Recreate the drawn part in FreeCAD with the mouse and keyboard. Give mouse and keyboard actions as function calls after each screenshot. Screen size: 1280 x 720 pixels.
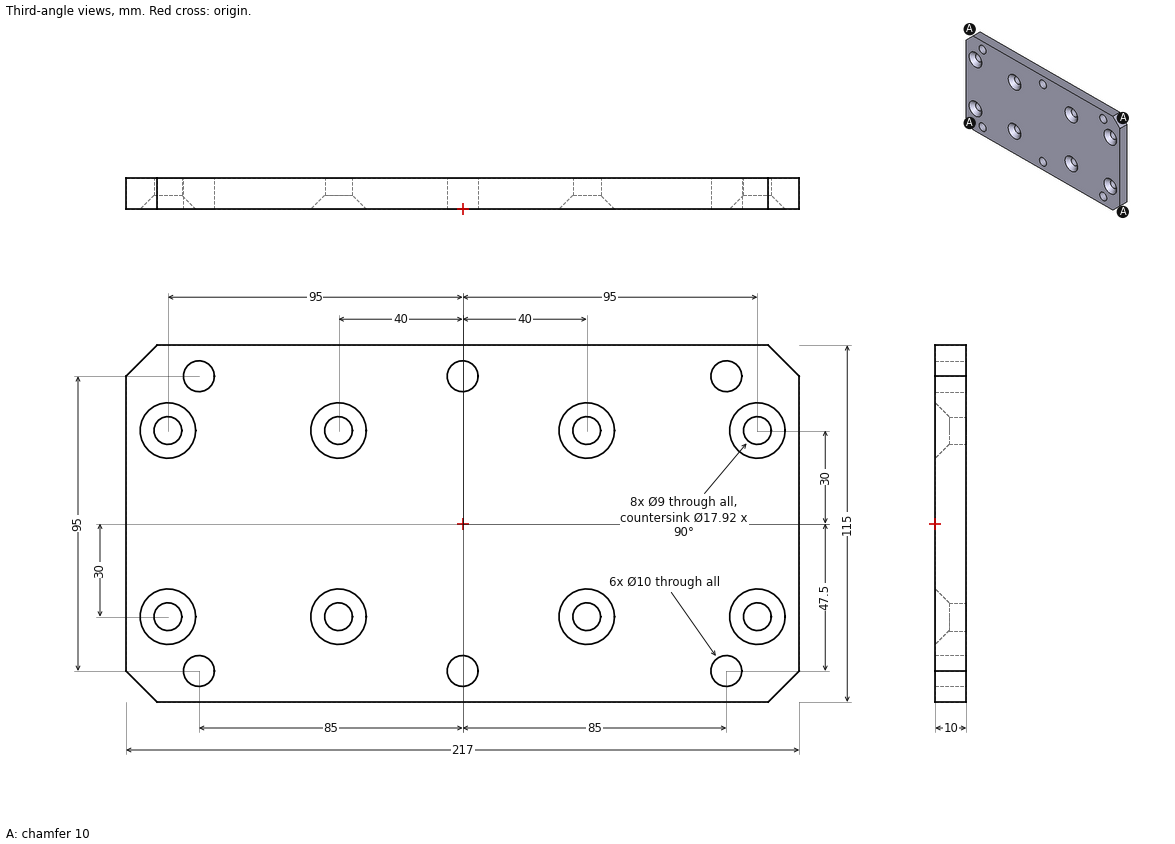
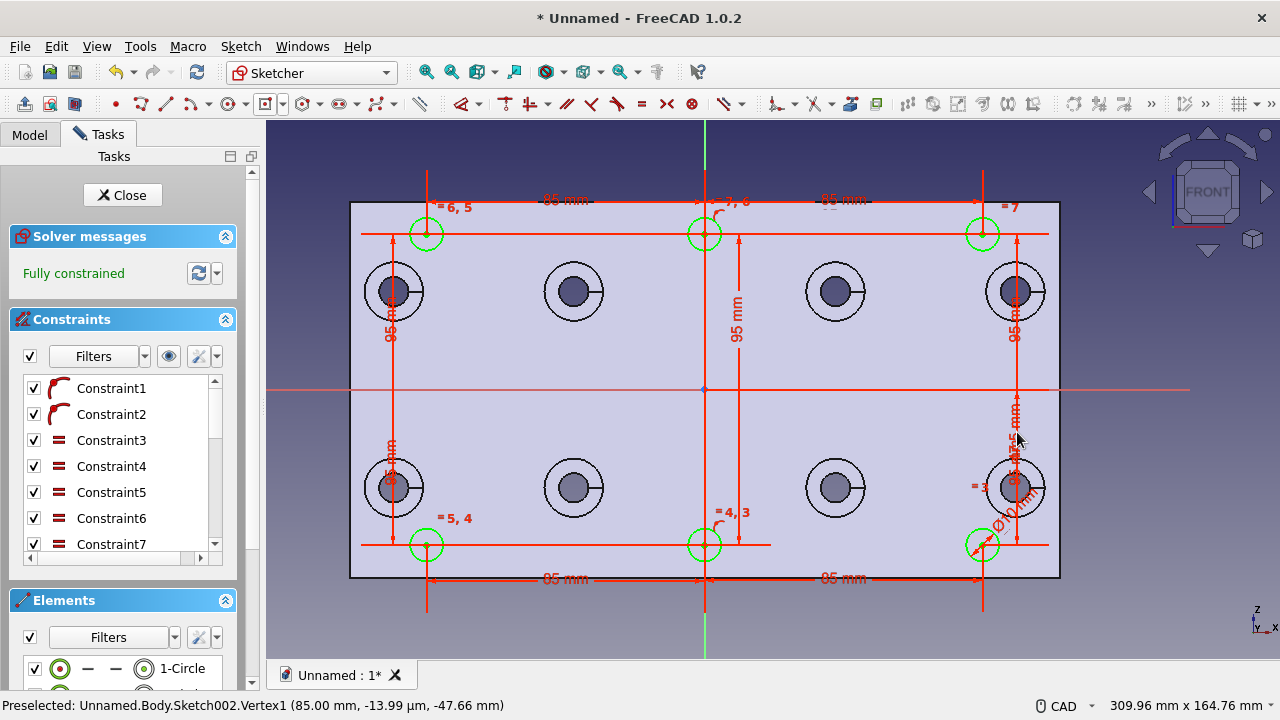
click(123, 195)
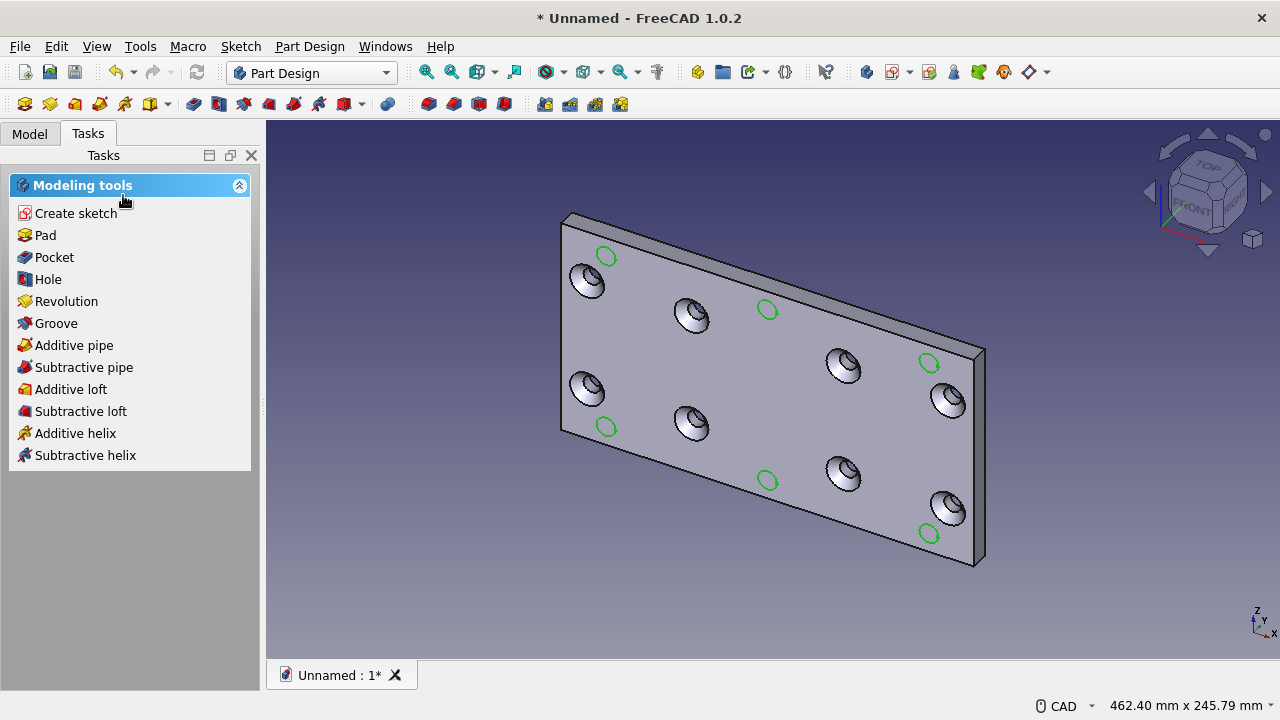
click(219, 104)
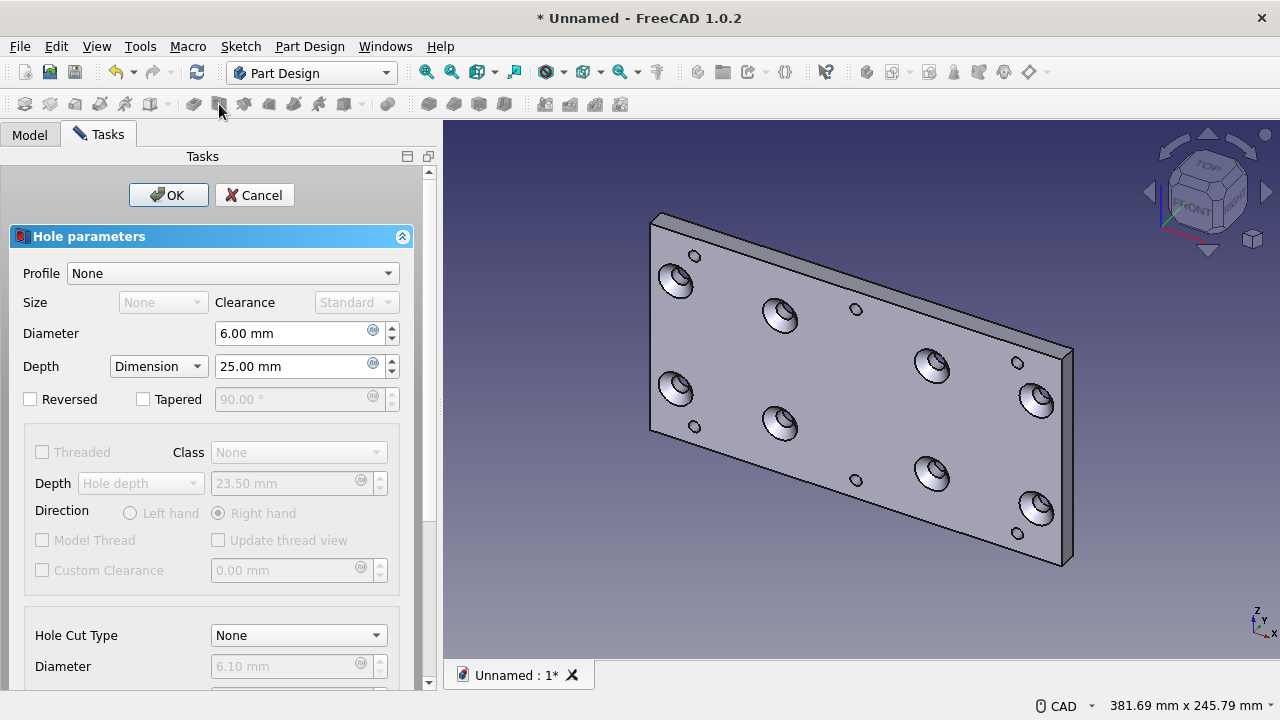
triple_click(300, 334)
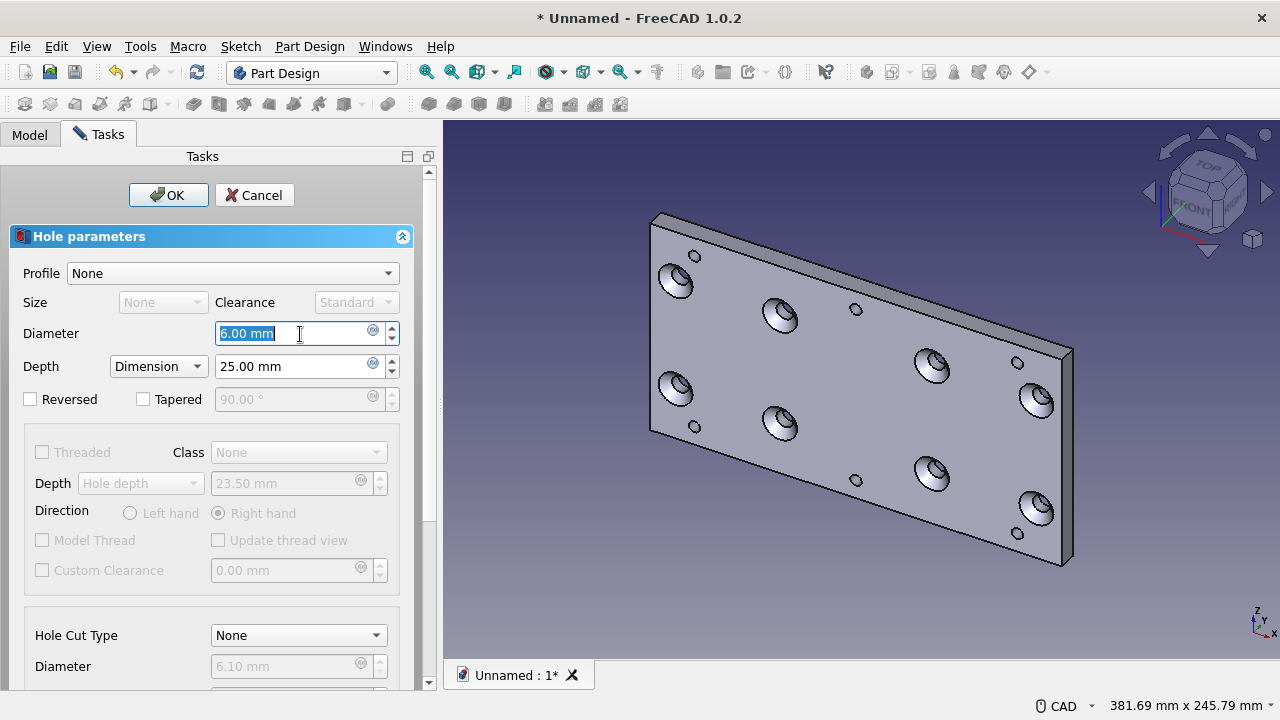
text(10)
key(Tab)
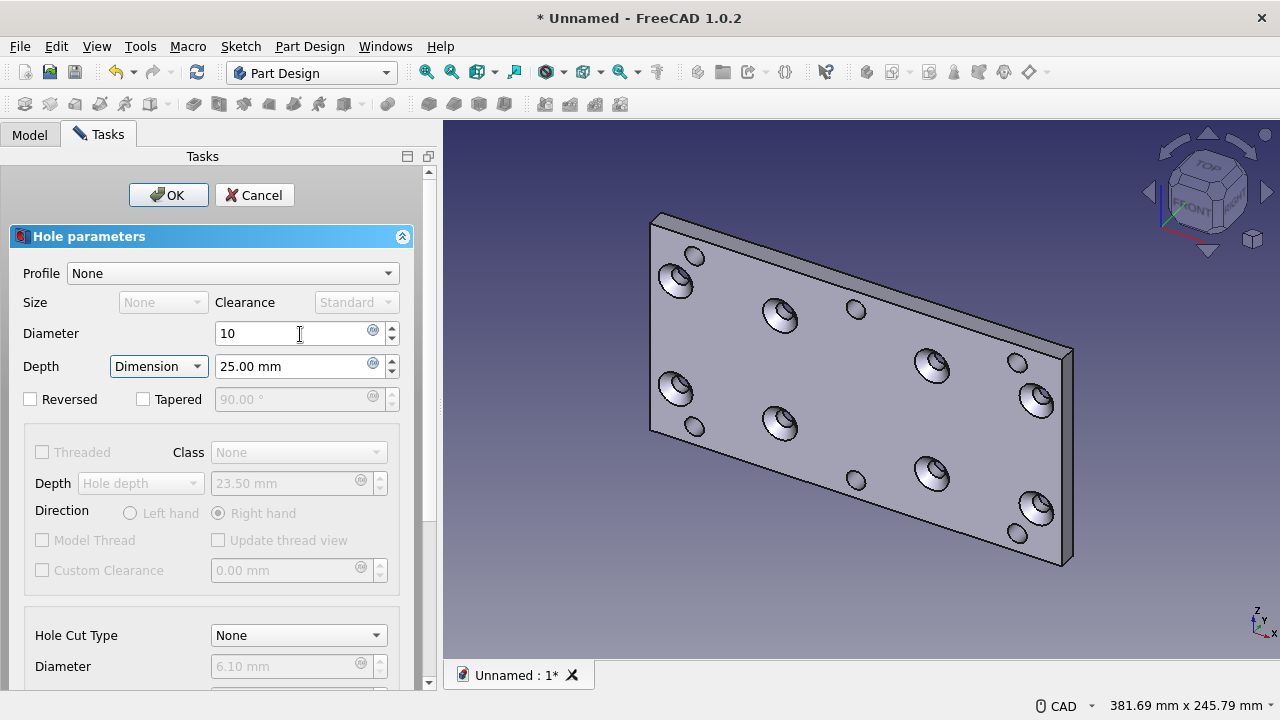
click(160, 366)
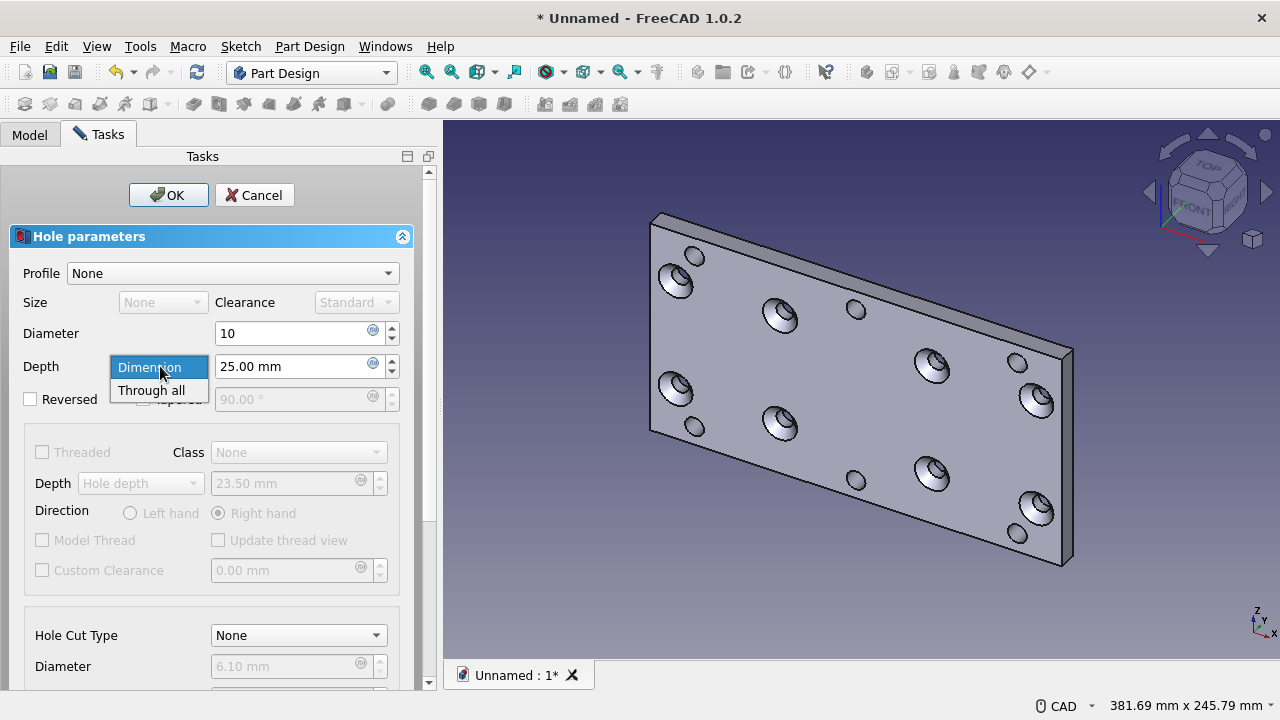
click(158, 390)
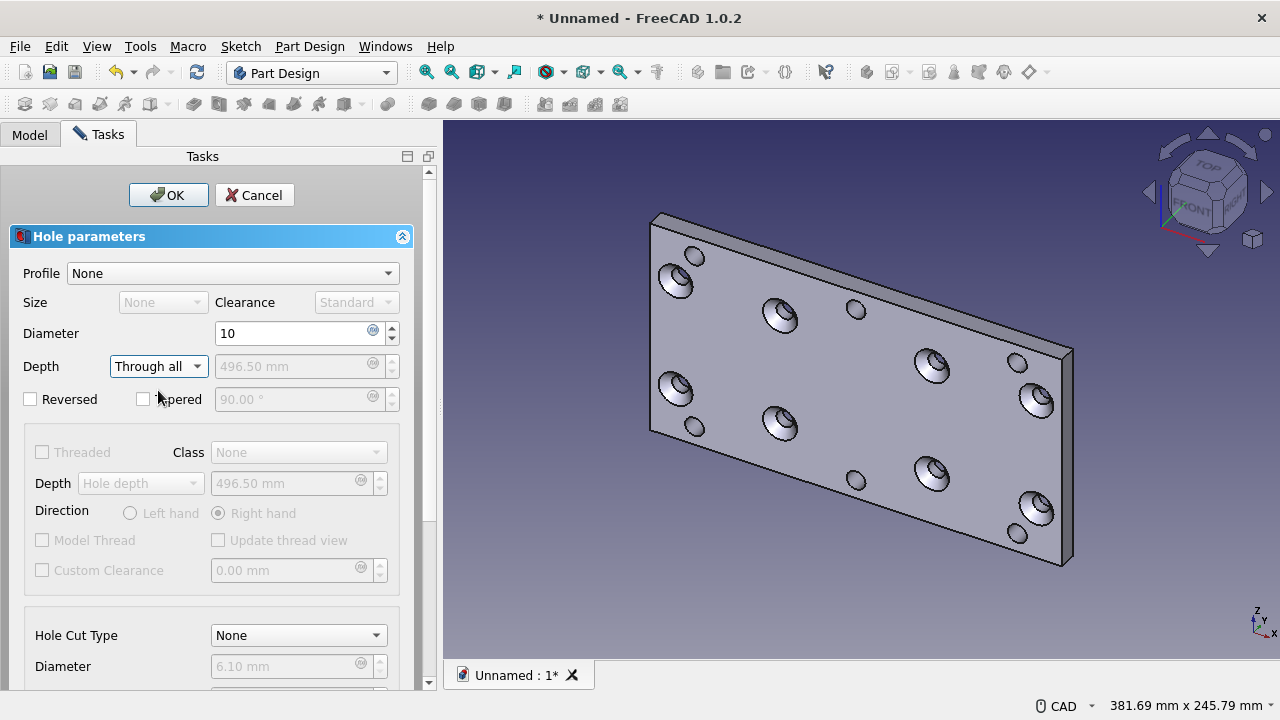
click(169, 195)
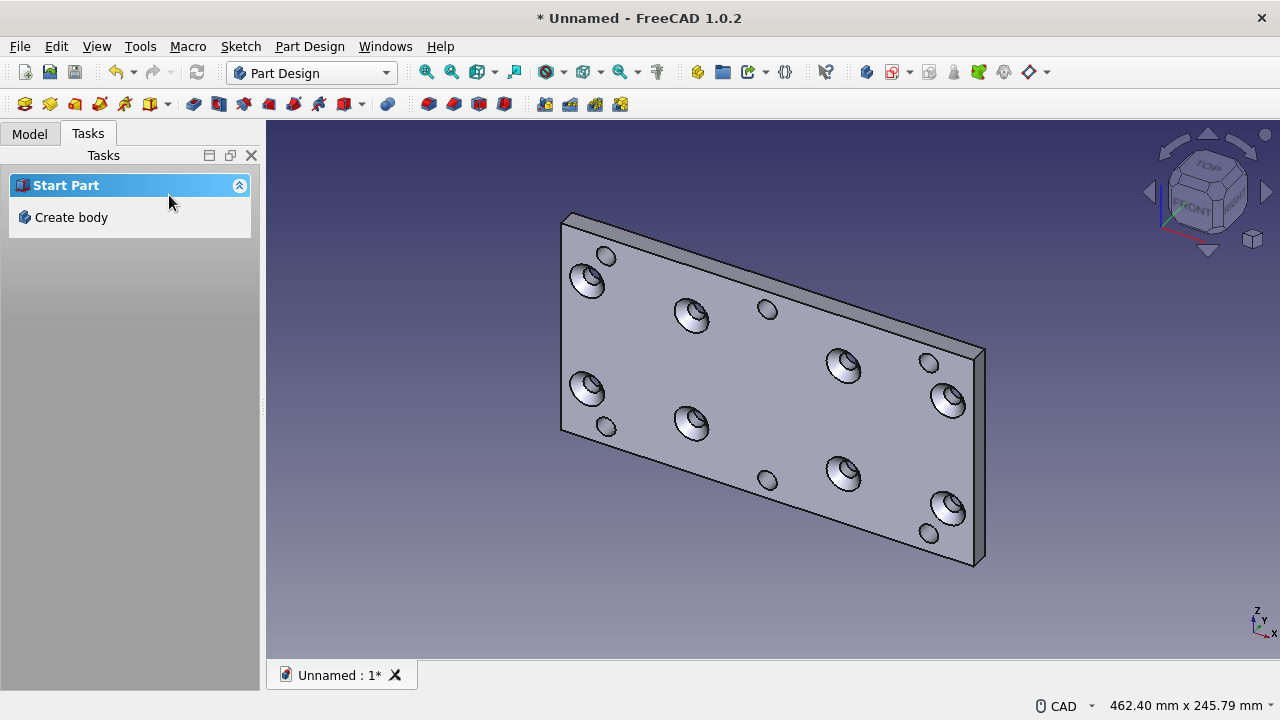
click(979, 353)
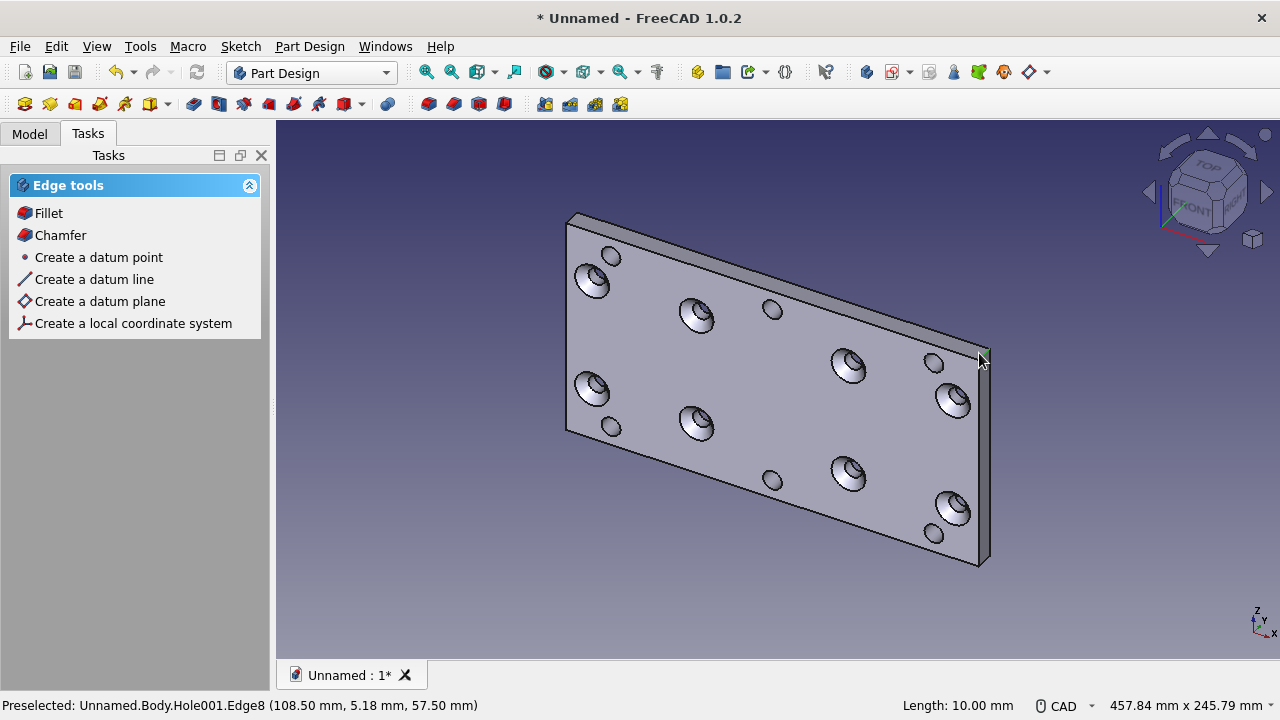
scroll(572, 217, up, 4)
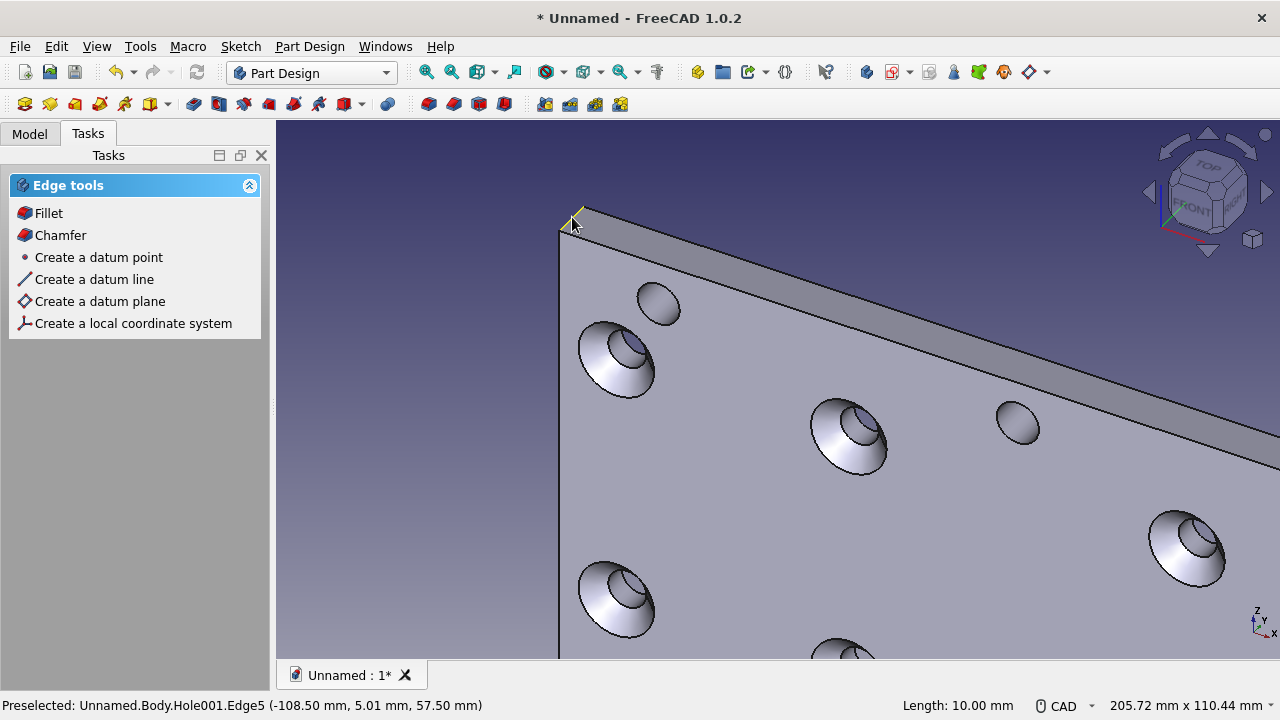
click(427, 72)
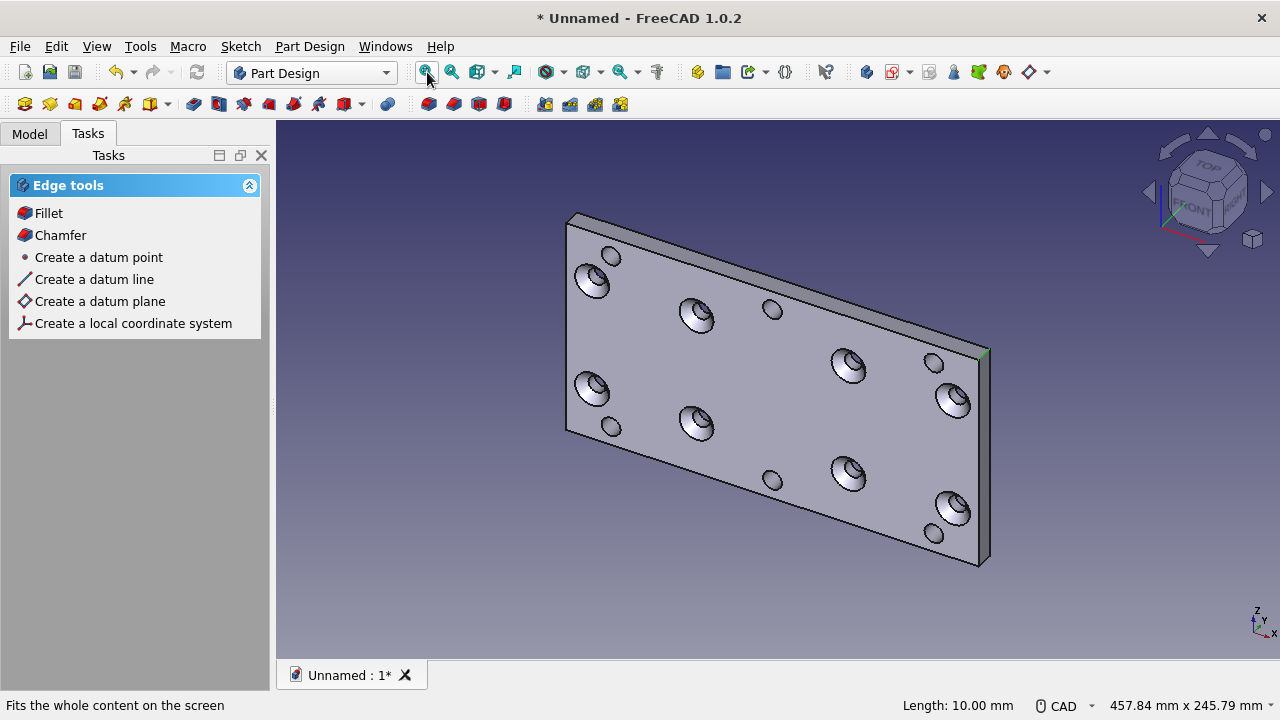
key(0)